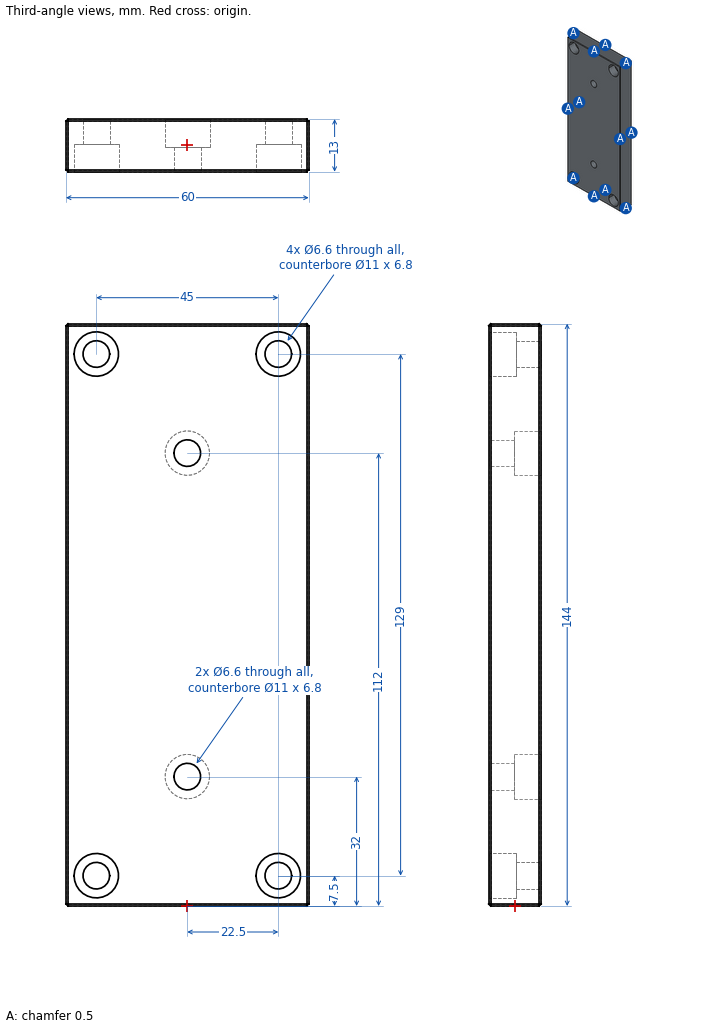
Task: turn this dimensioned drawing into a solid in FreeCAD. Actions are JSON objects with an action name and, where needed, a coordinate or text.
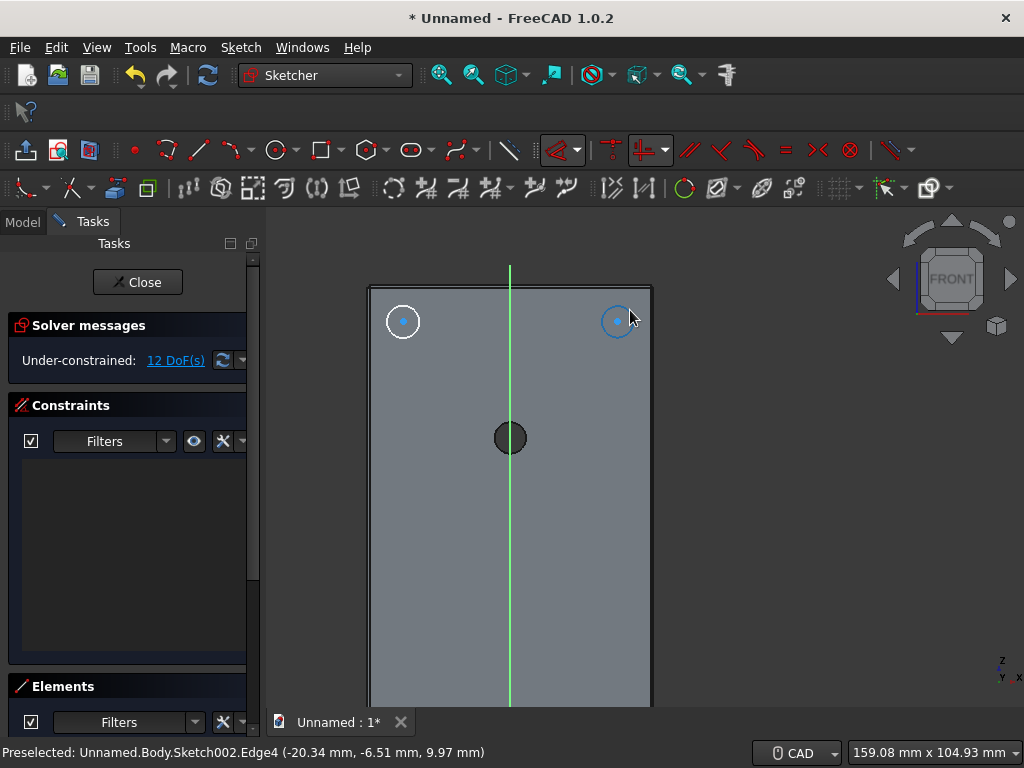
{"action": "left_click", "coordinate": [629, 311]}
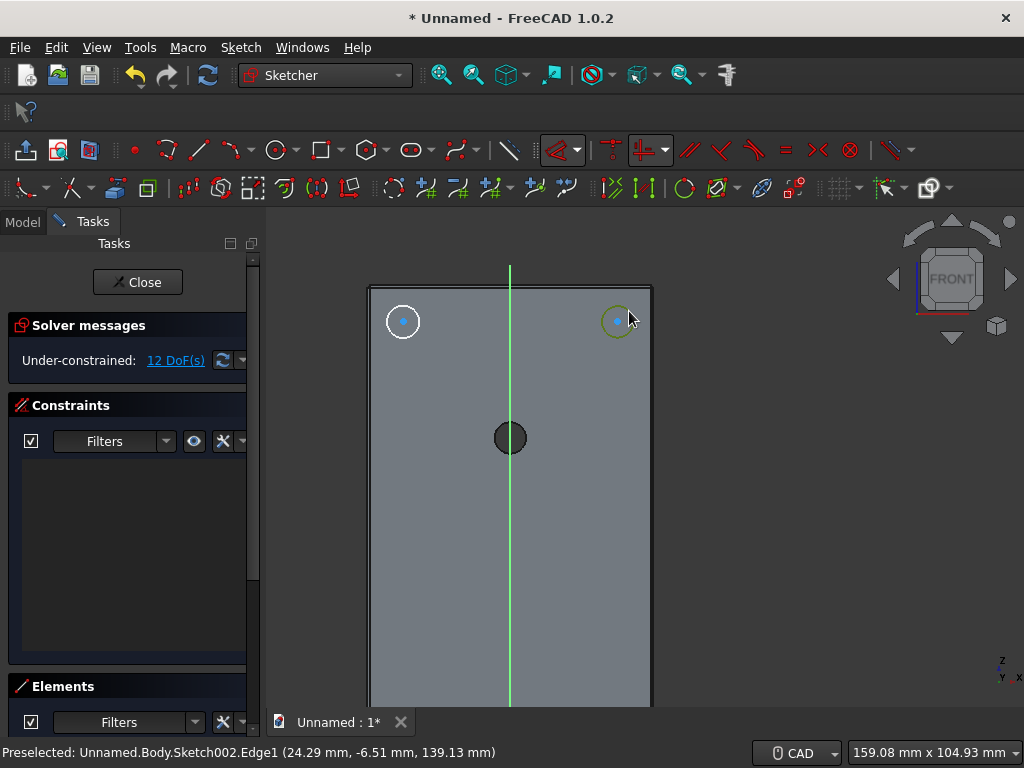
{"action": "left_click", "coordinate": [415, 310]}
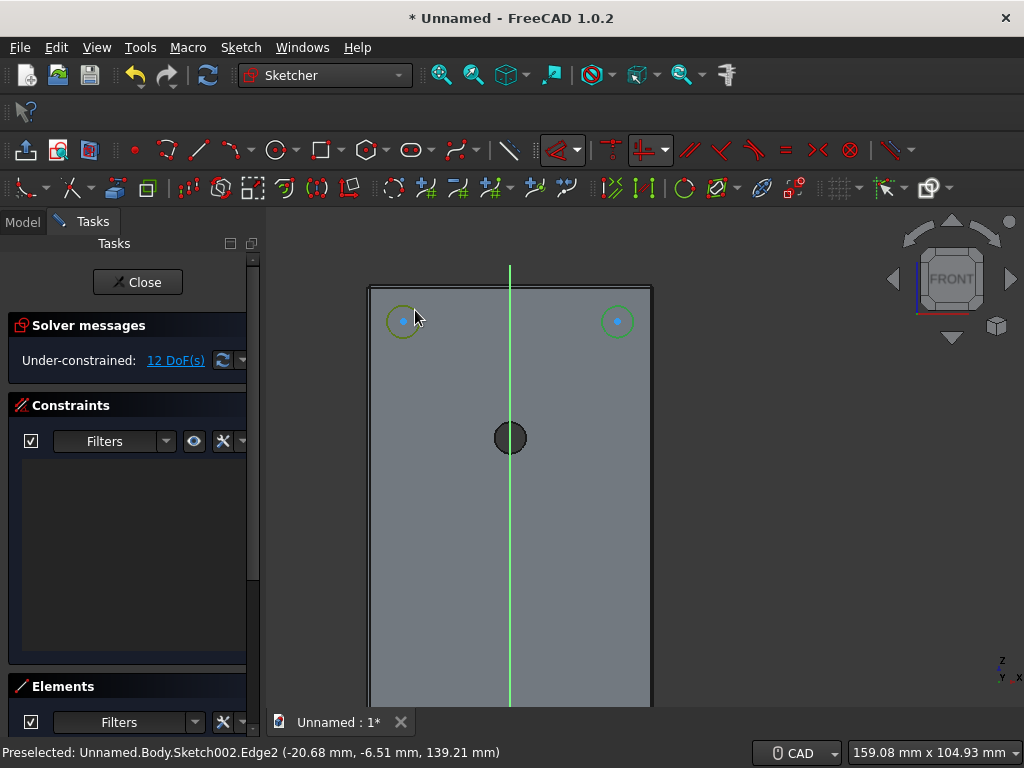
{"action": "scroll", "coordinate": [630, 309], "scroll_direction": "down", "scroll_amount": 4}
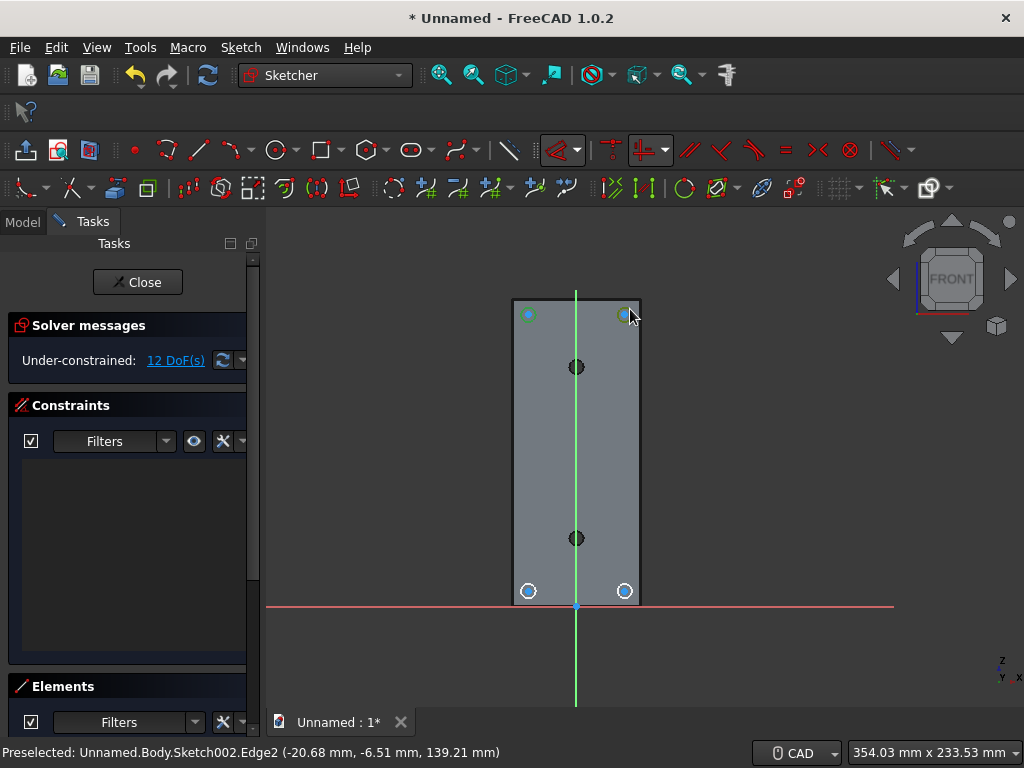
{"action": "scroll", "coordinate": [630, 586], "scroll_direction": "up", "scroll_amount": 4}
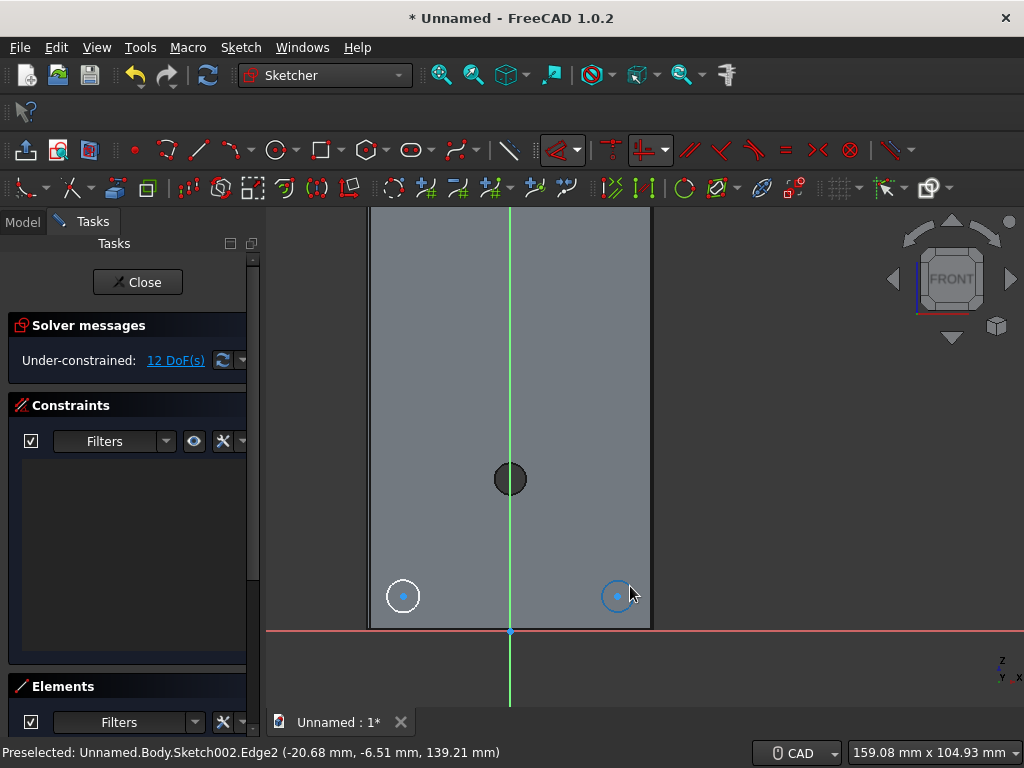
{"action": "left_click", "coordinate": [629, 585]}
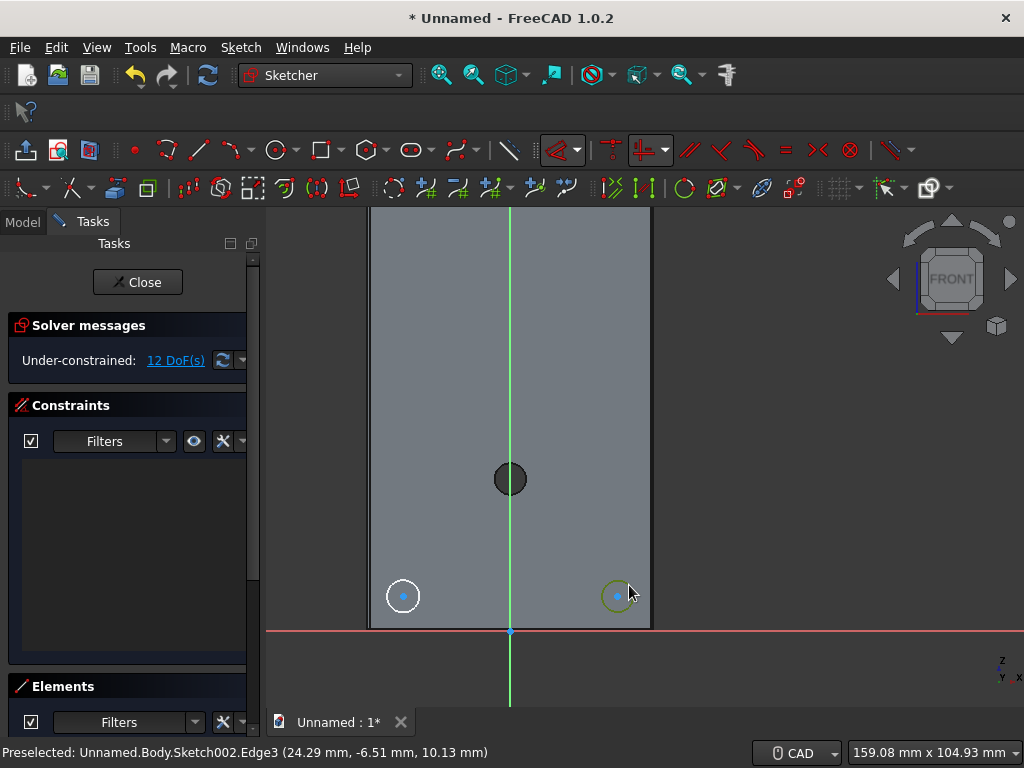
{"action": "left_click", "coordinate": [415, 585]}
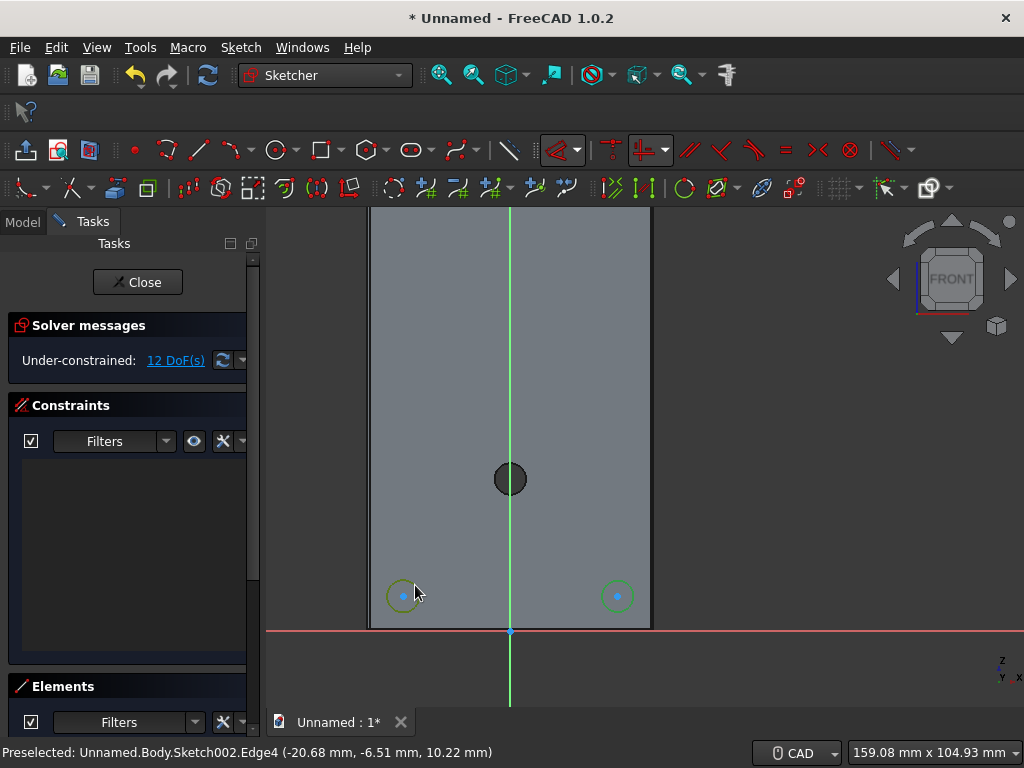
{"action": "key", "text": "e"}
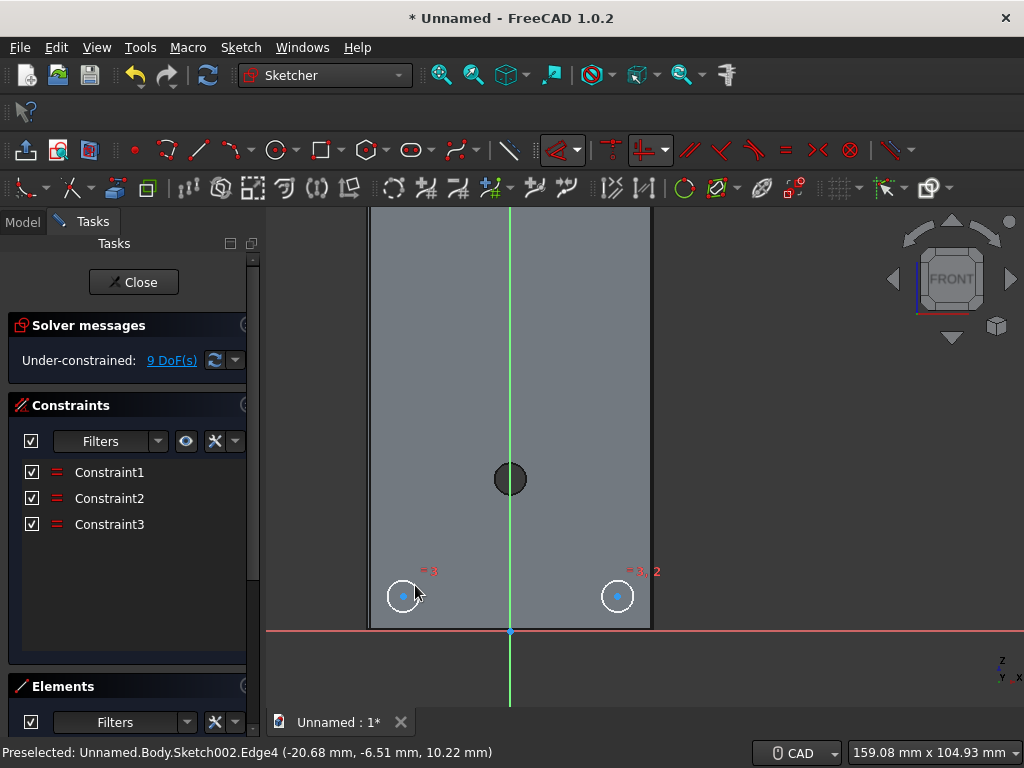
{"action": "scroll", "coordinate": [630, 586], "scroll_direction": "down", "scroll_amount": 4}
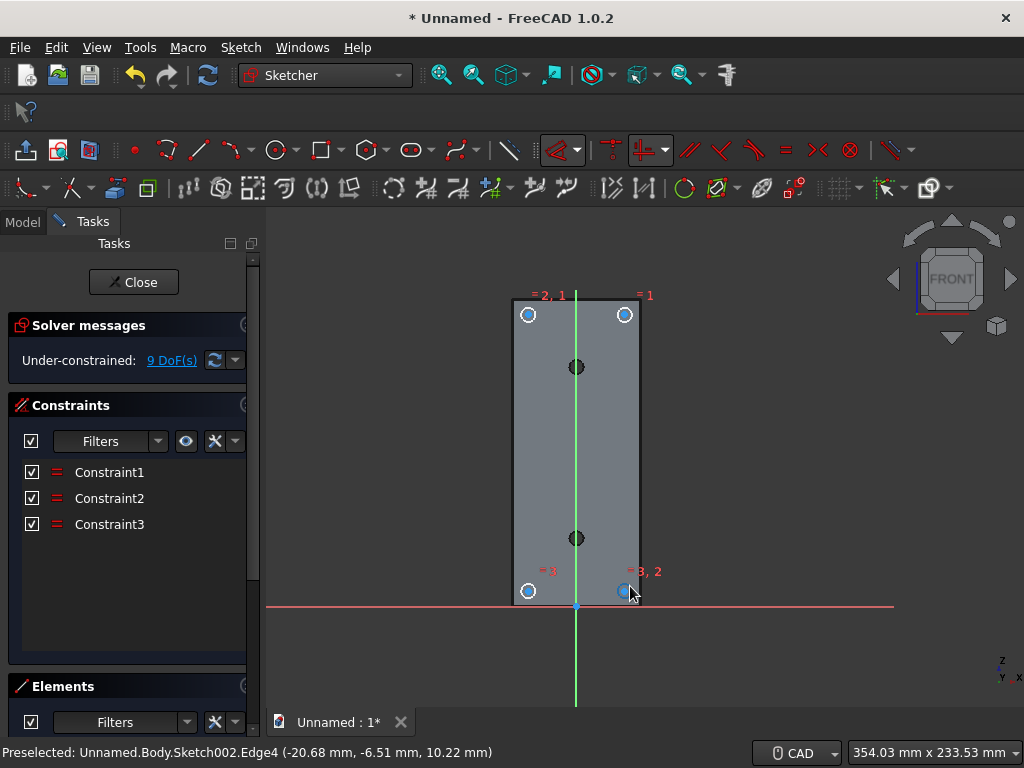
{"action": "scroll", "coordinate": [630, 310], "scroll_direction": "up", "scroll_amount": 6}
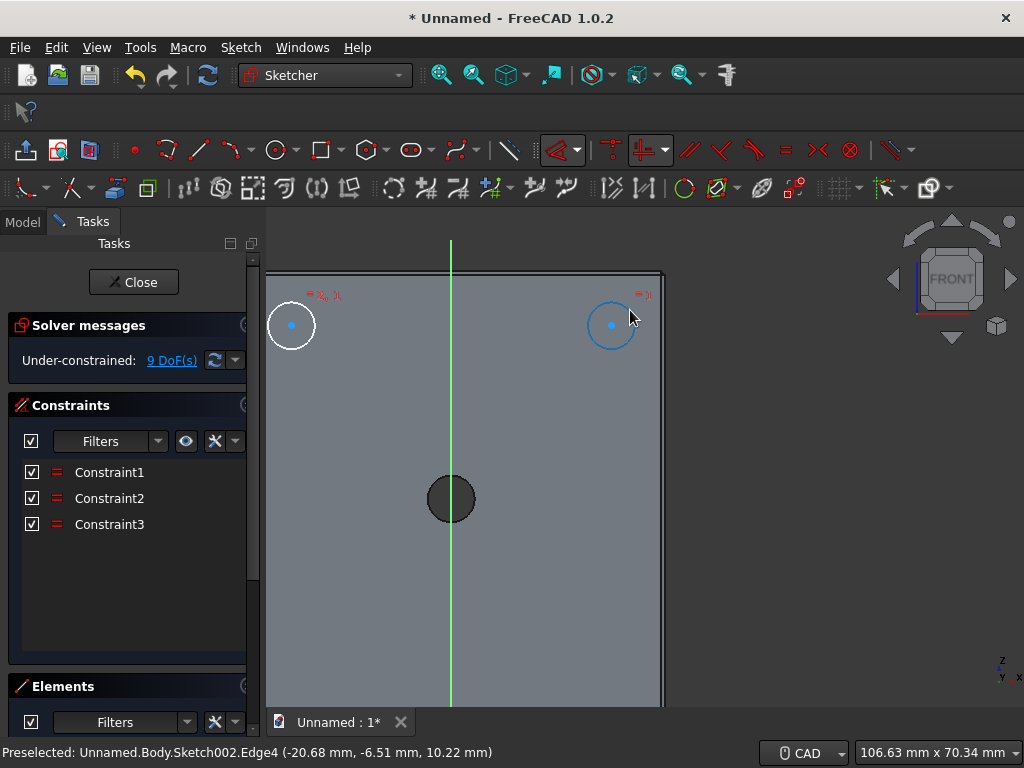
{"action": "left_click", "coordinate": [628, 309]}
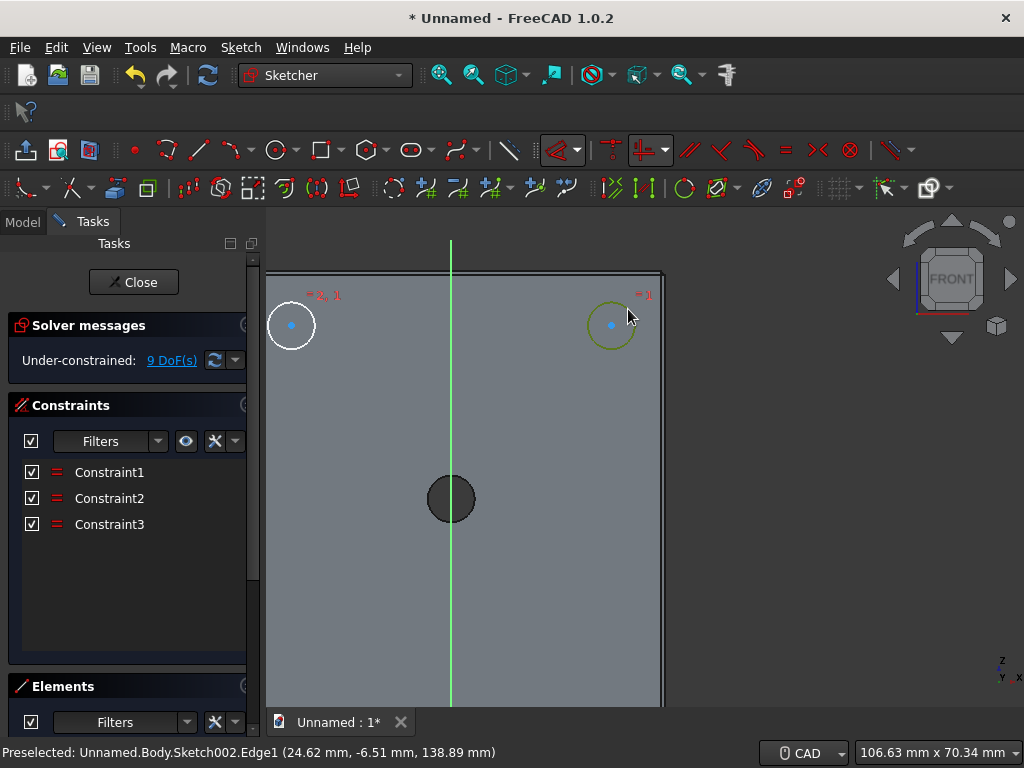
{"action": "key", "text": "k o"}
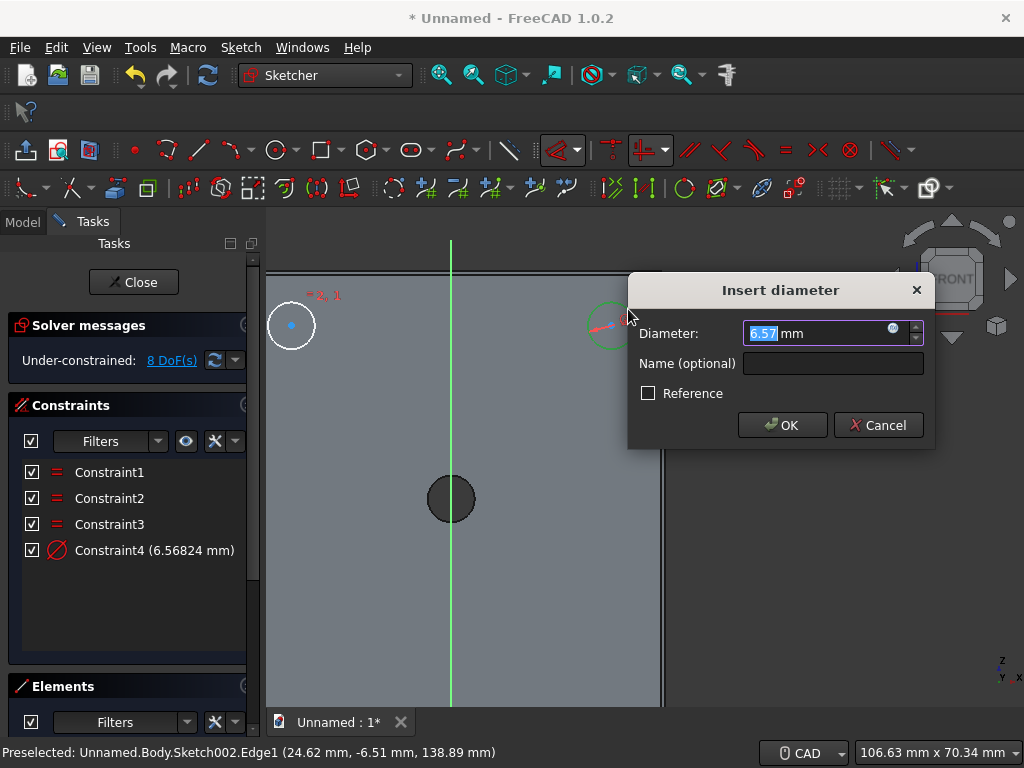
{"action": "type", "text": "6.6"}
{"action": "key", "text": "Return"}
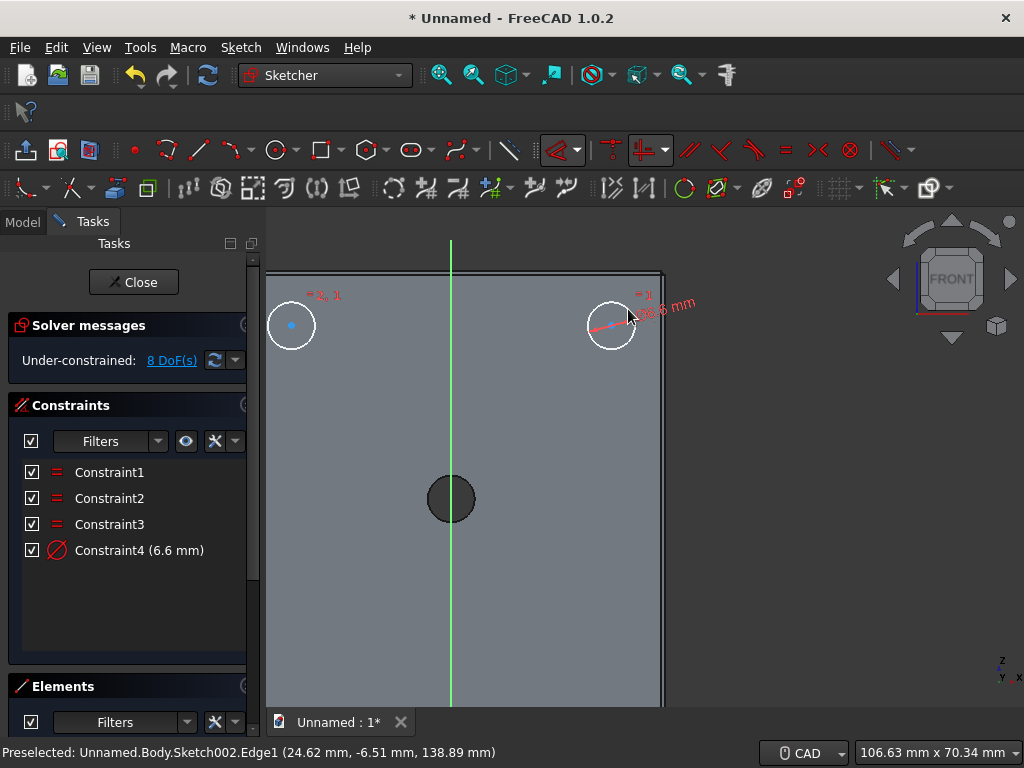
{"action": "scroll", "coordinate": [630, 310], "scroll_direction": "down", "scroll_amount": 6}